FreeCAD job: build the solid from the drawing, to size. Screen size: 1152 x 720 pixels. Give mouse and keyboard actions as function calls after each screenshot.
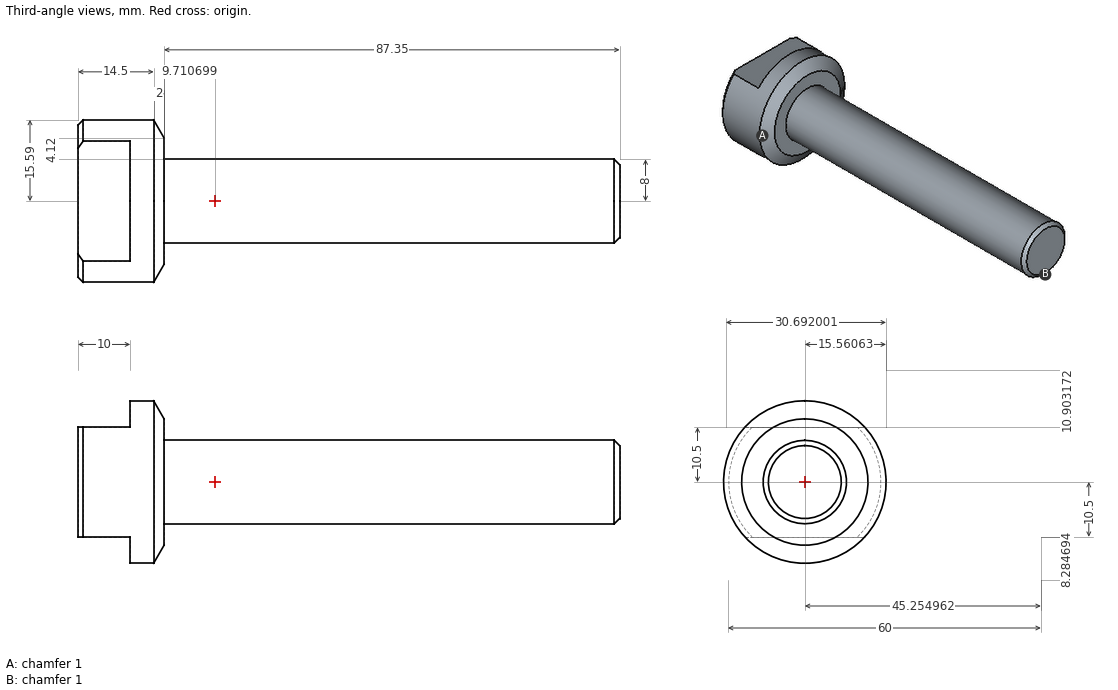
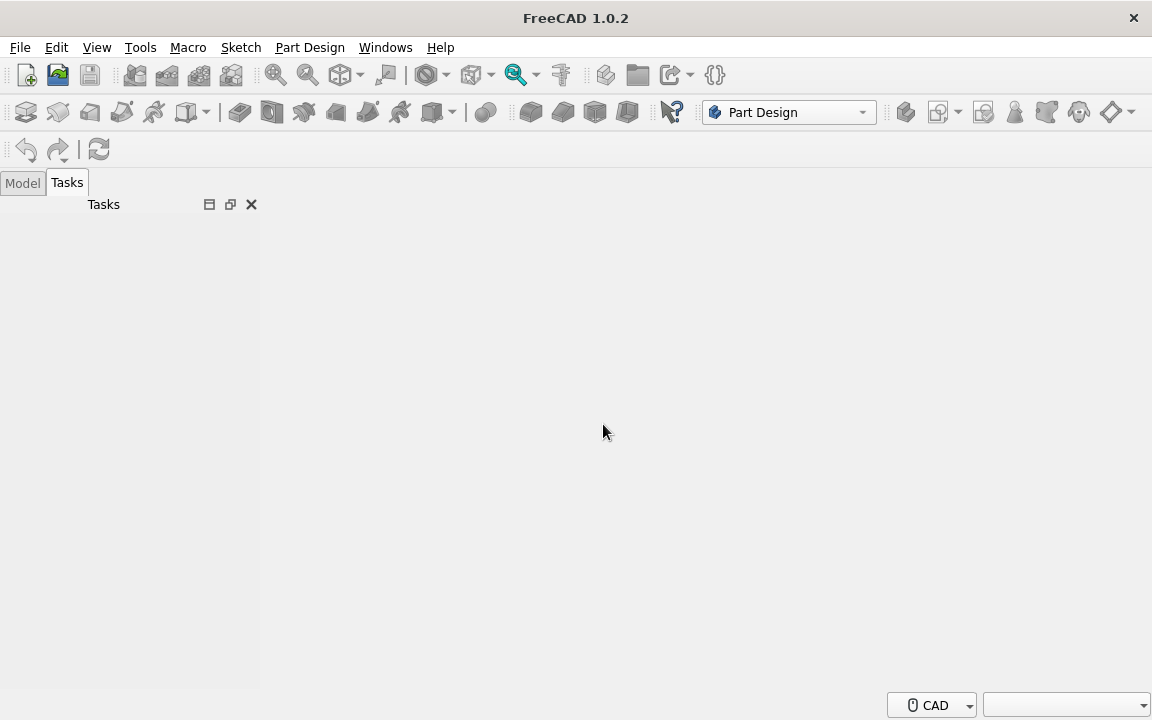
click(26, 76)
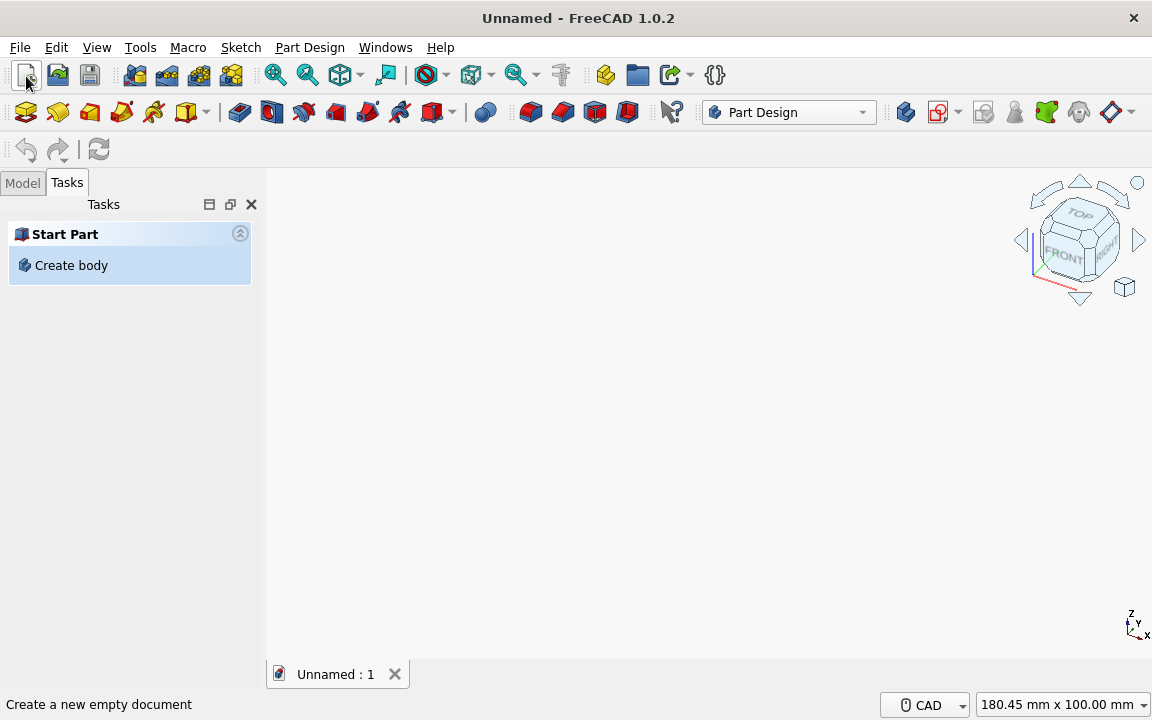
click(938, 112)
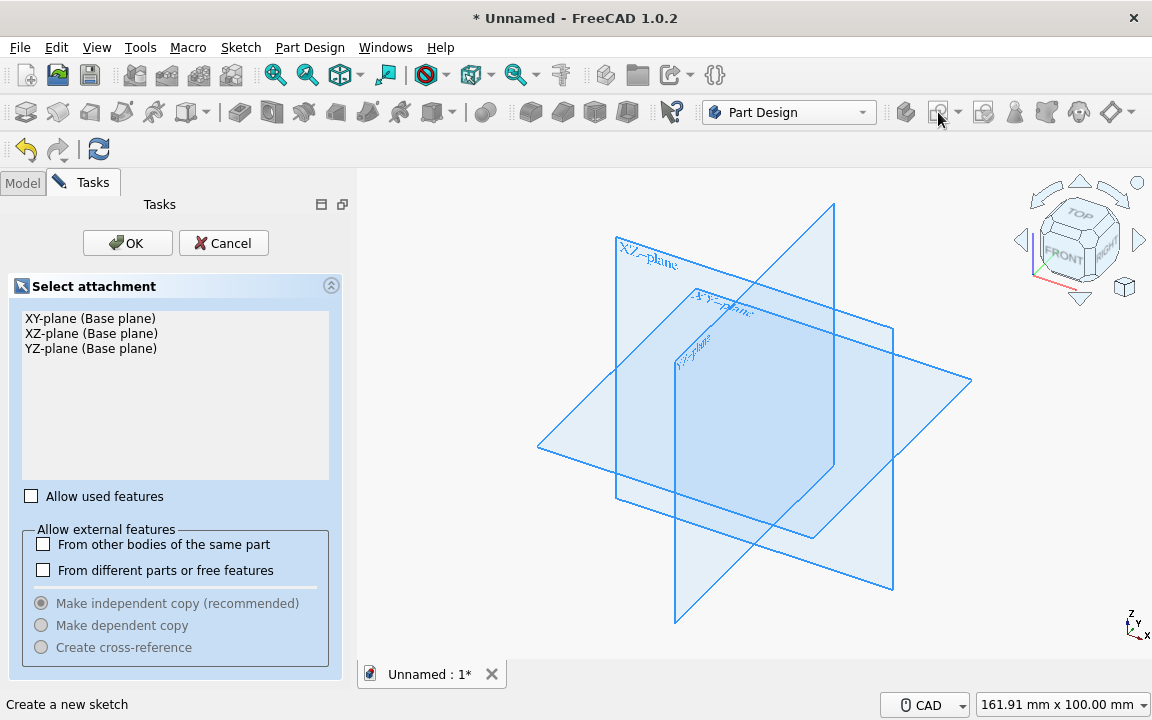
click(82, 318)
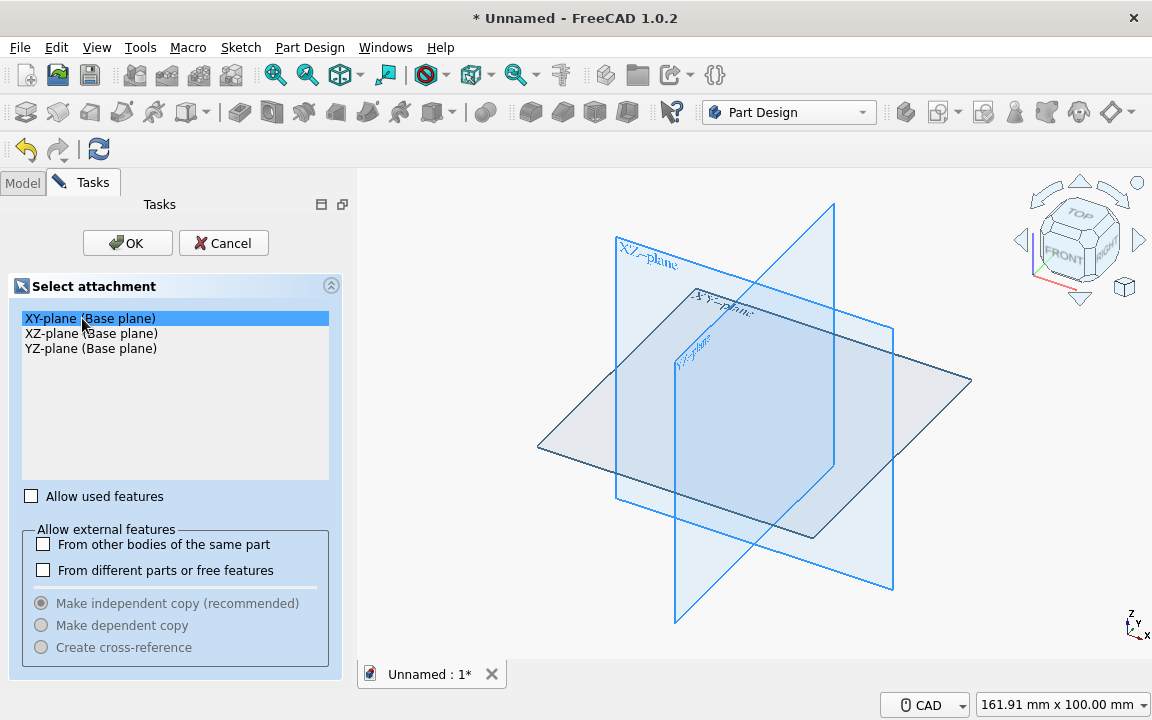
click(128, 243)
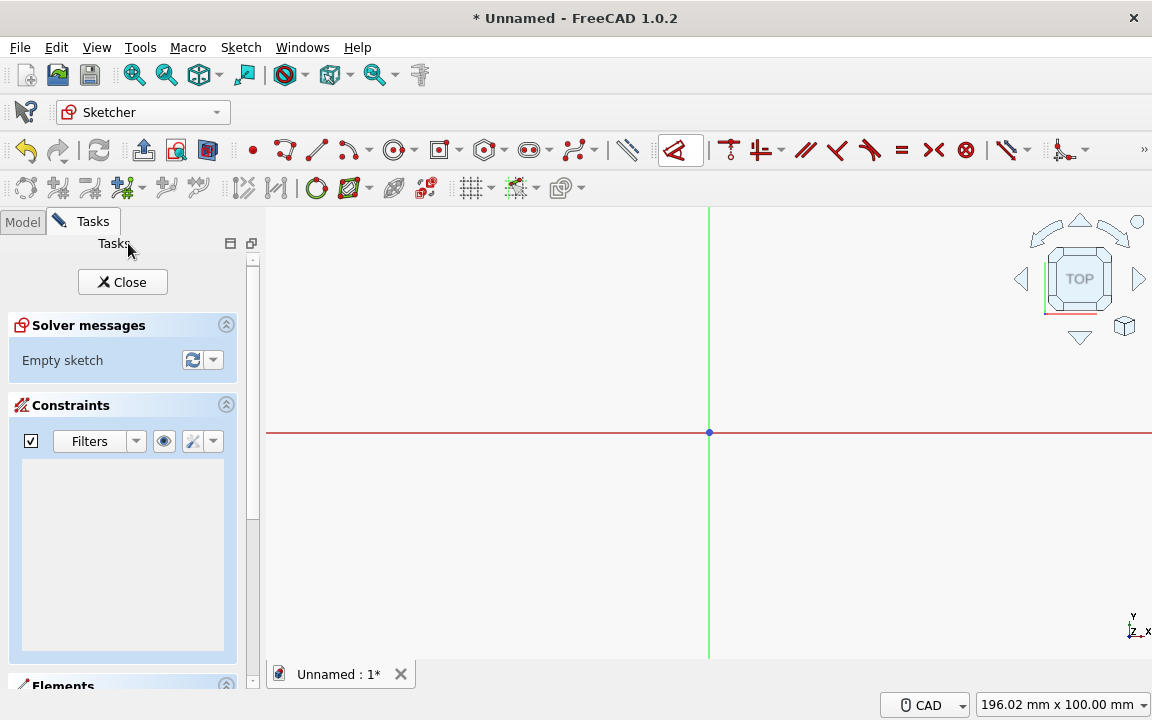
scroll(294, 592, down, 1)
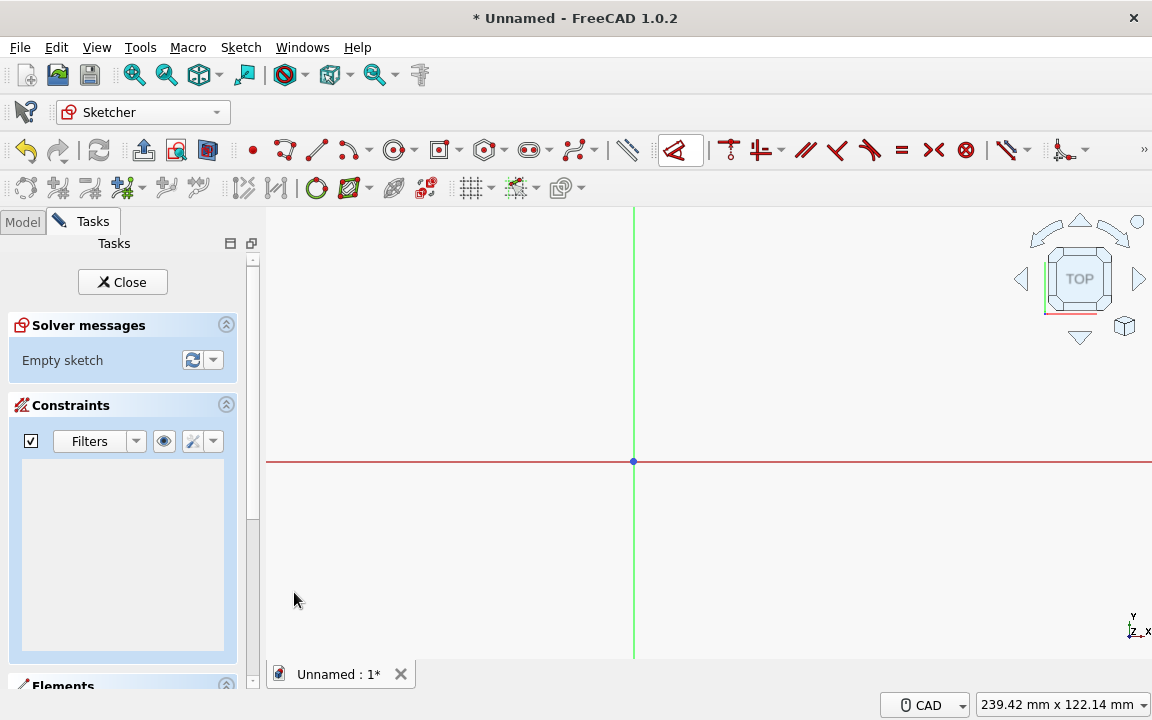
click(286, 150)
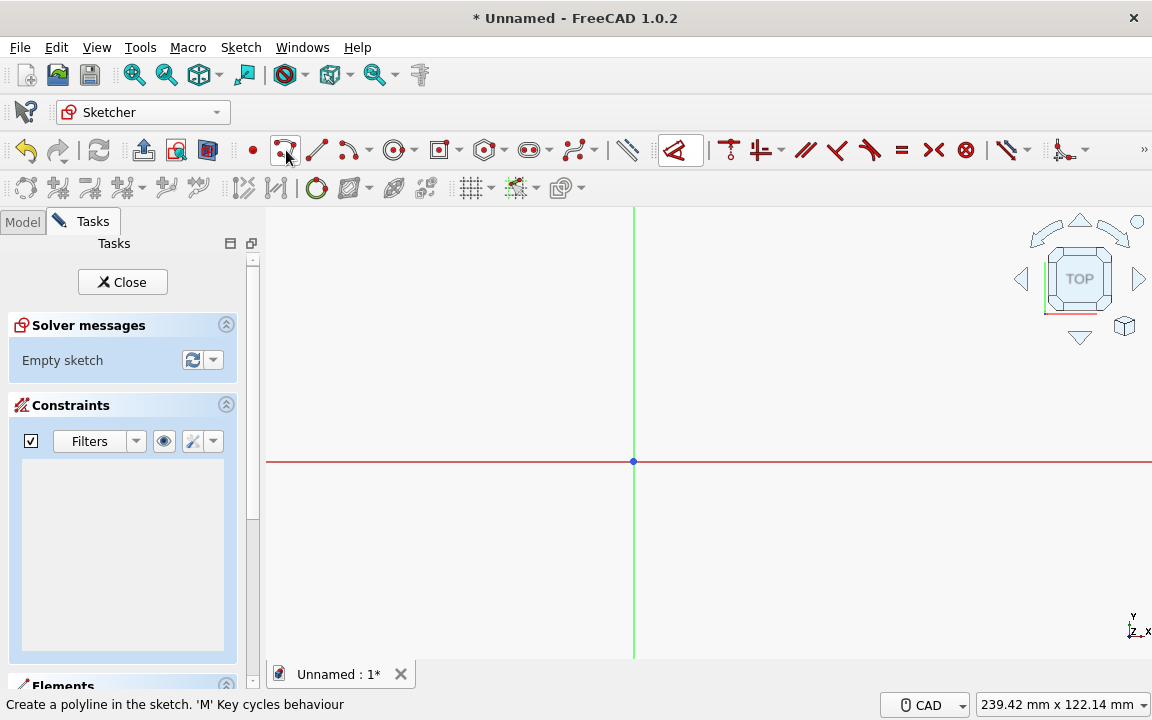
click(598, 432)
click(598, 417)
click(590, 404)
click(537, 404)
click(537, 462)
click(921, 453)
click(921, 432)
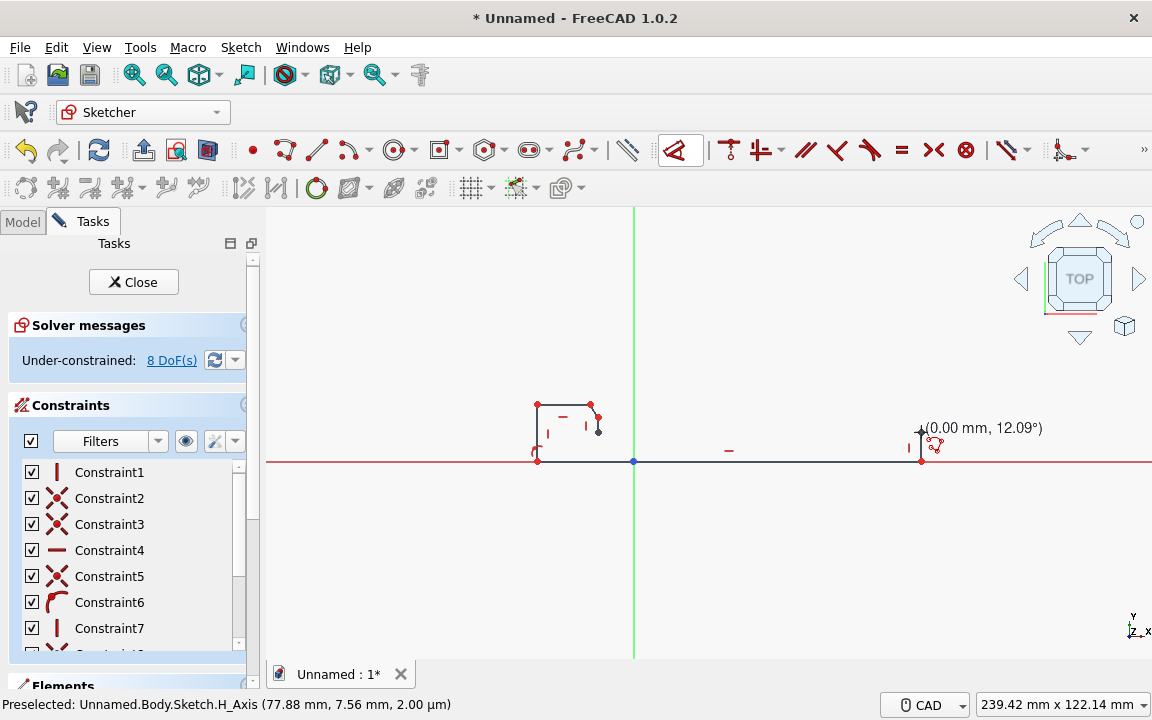
scroll(598, 432, up, 4)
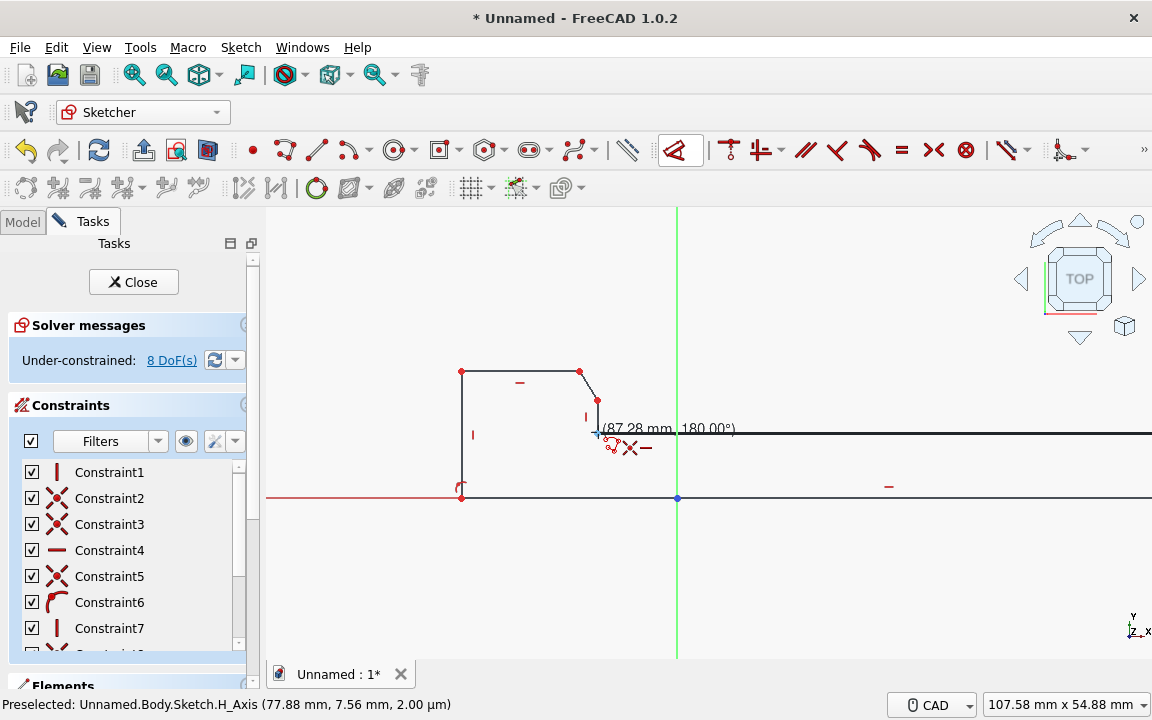
click(598, 434)
key(Escape)
key(Escape)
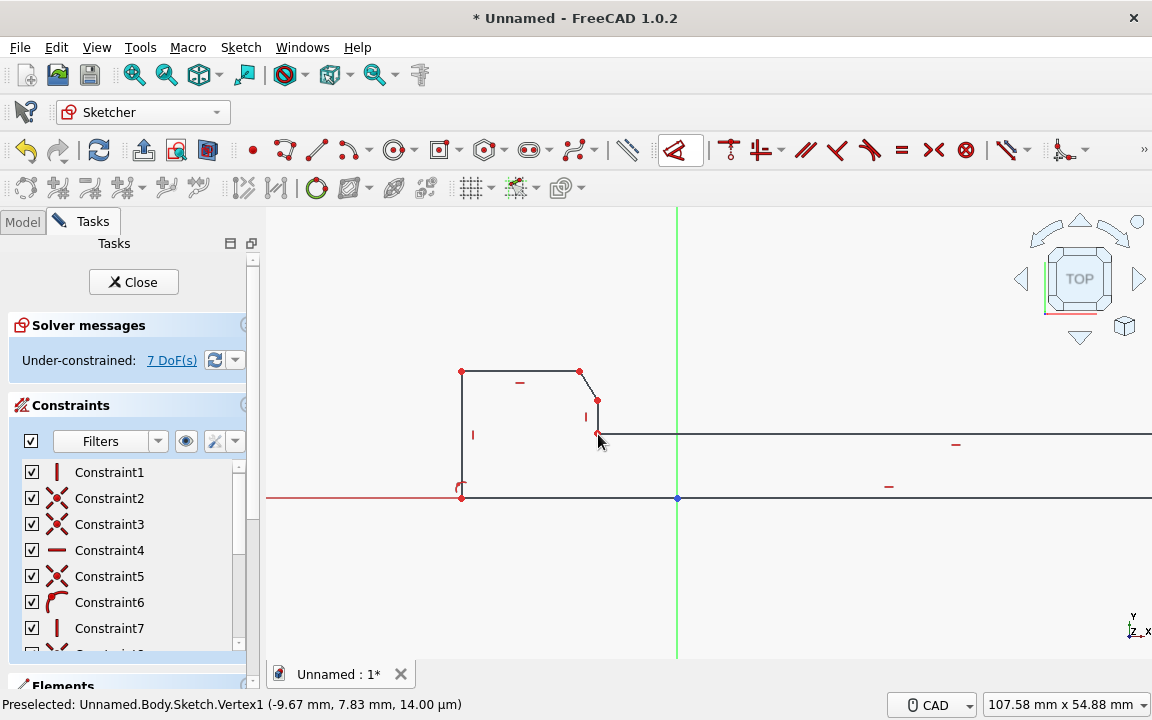
scroll(338, 432, down, 3)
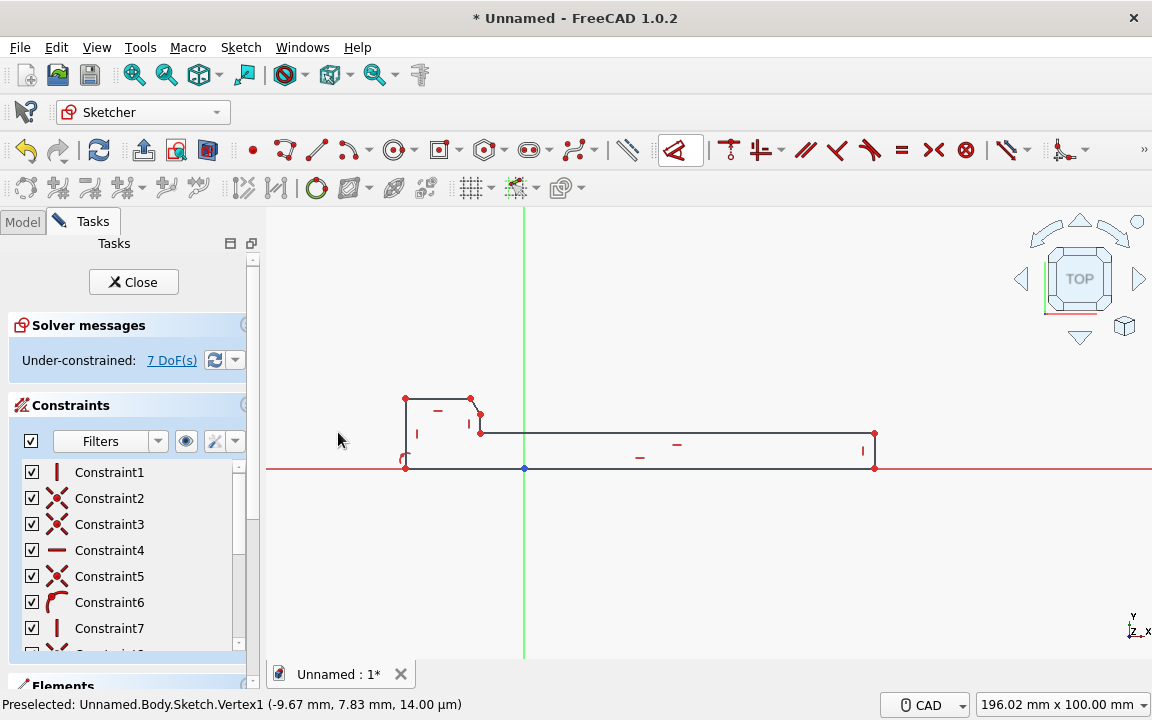
scroll(875, 458, up, 2)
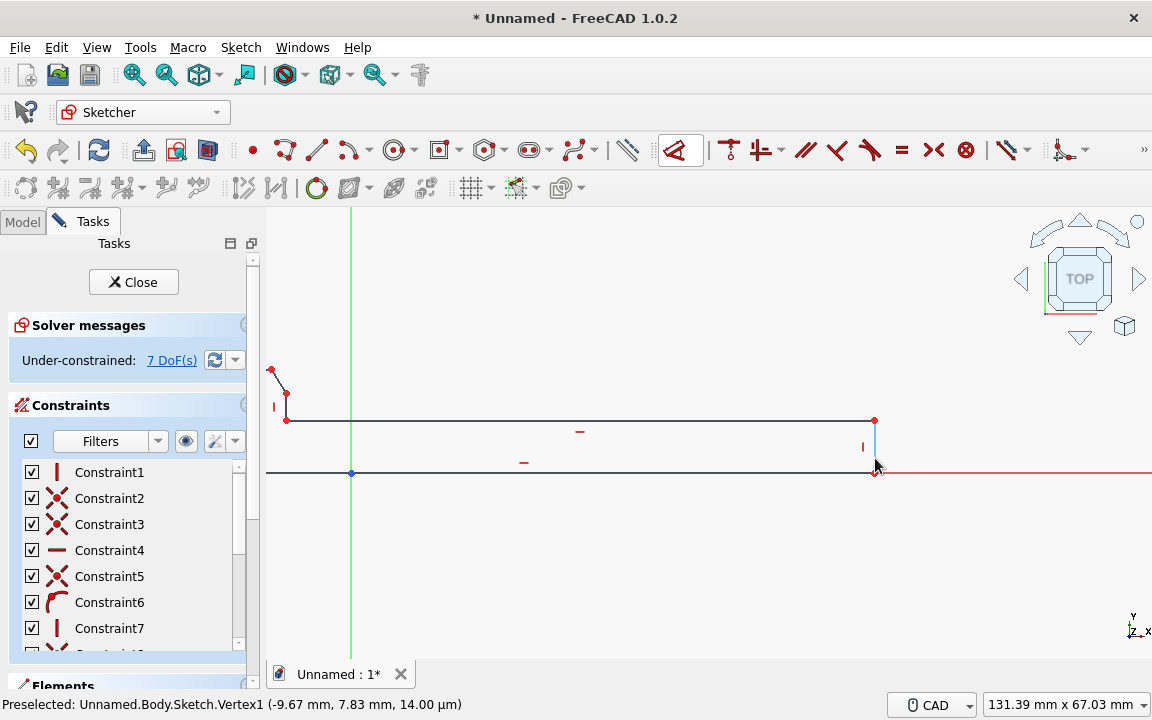
click(875, 458)